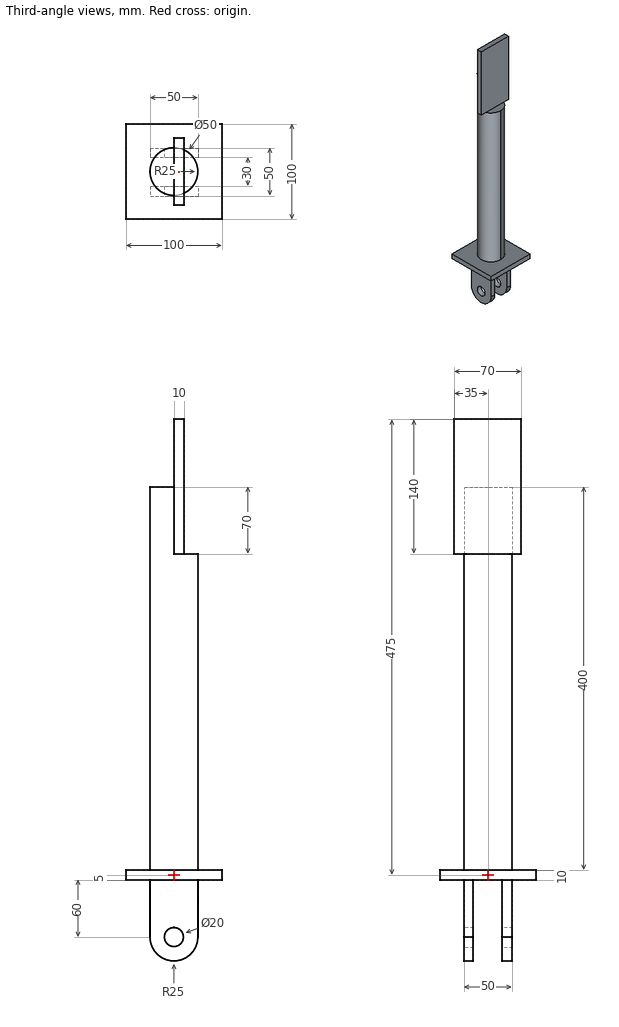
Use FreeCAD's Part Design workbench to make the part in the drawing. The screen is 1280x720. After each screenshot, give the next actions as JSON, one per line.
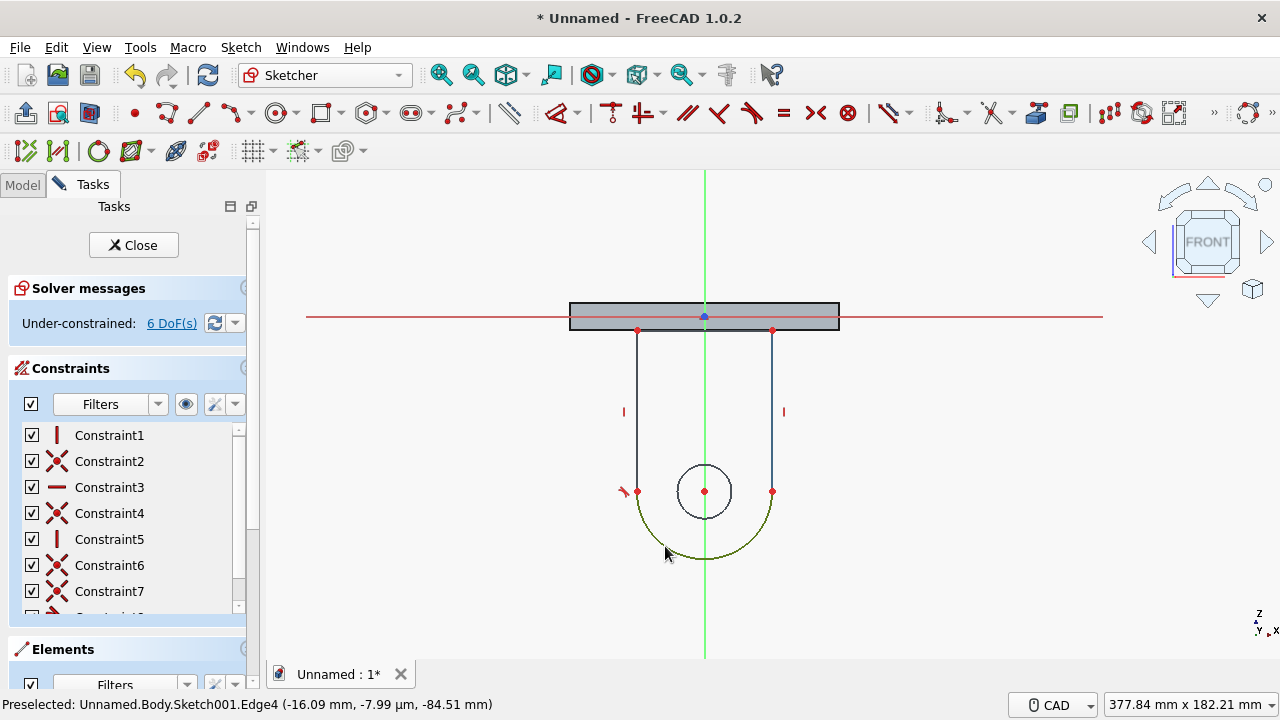
{"action": "key", "text": "t"}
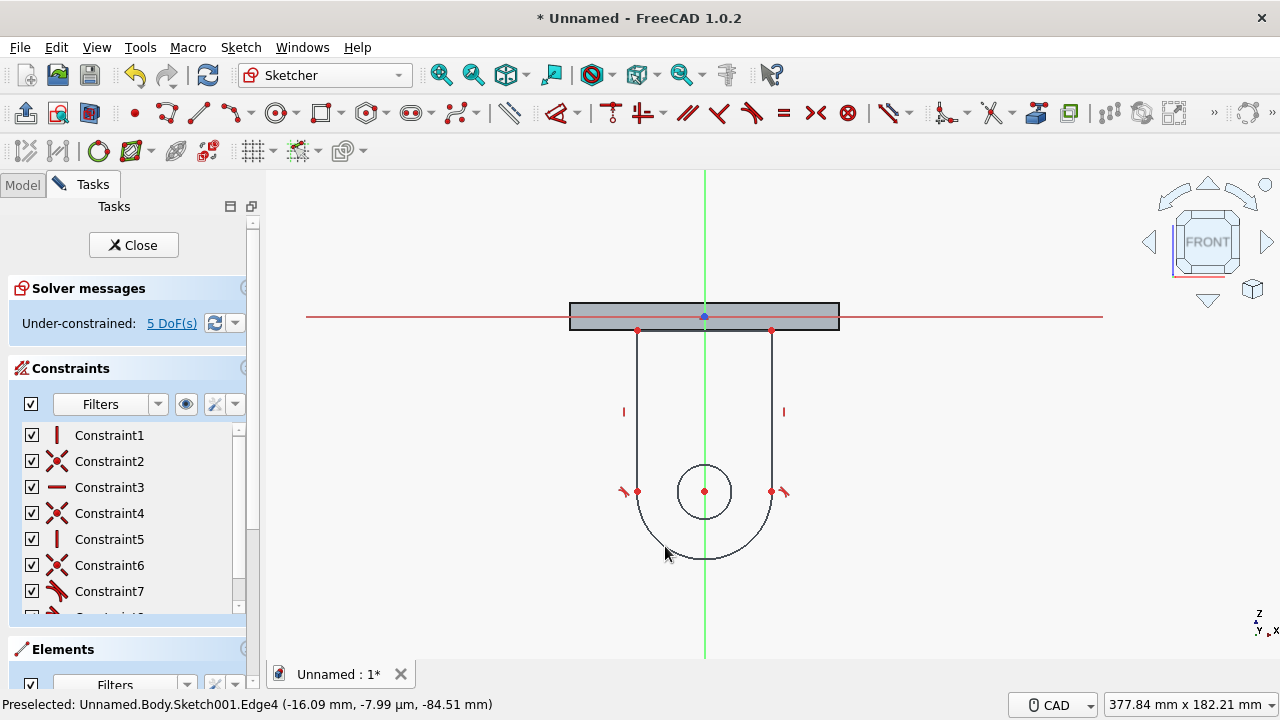
{"action": "left_click", "coordinate": [704, 492]}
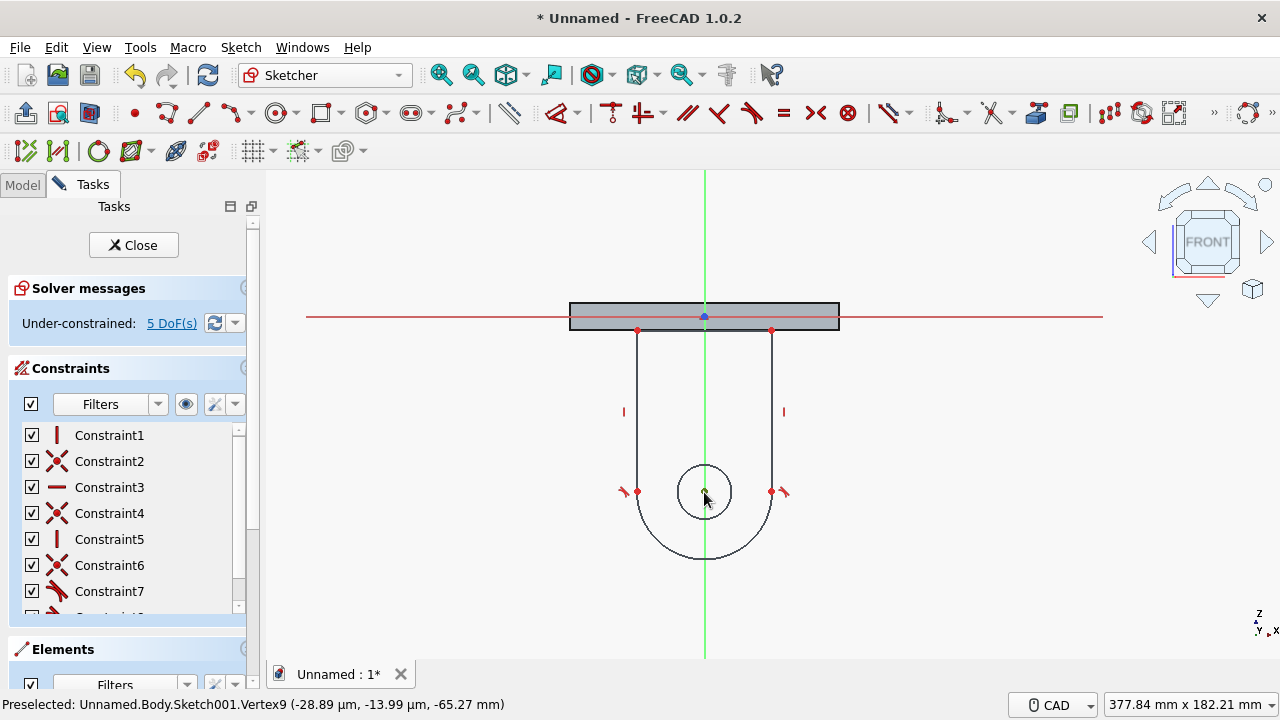
{"action": "left_click", "coordinate": [705, 600]}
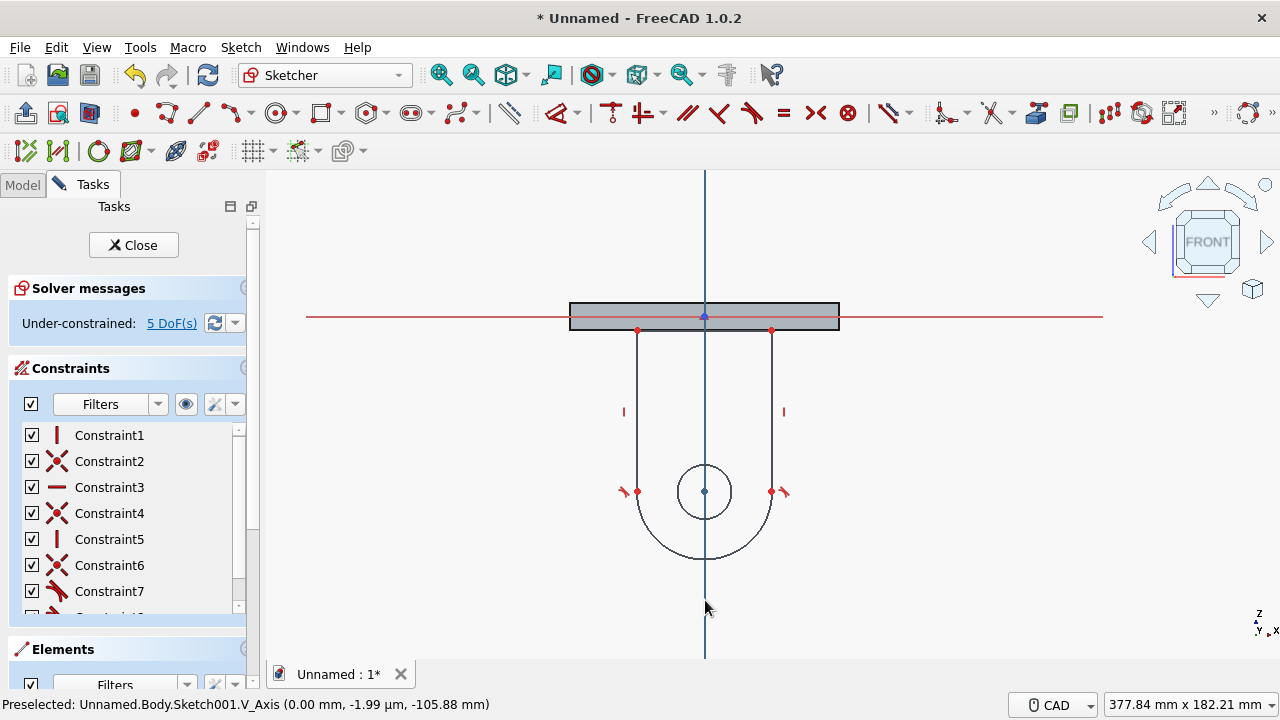
{"action": "key", "text": "c"}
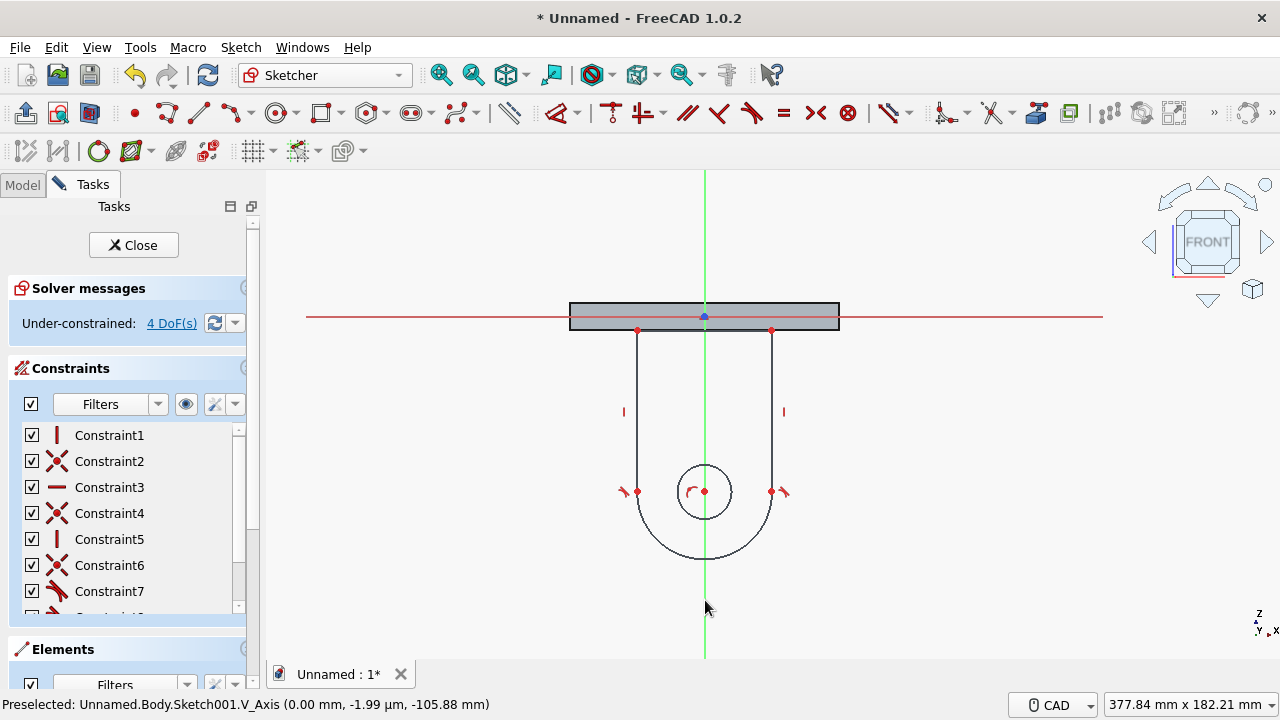
{"action": "key", "text": "d"}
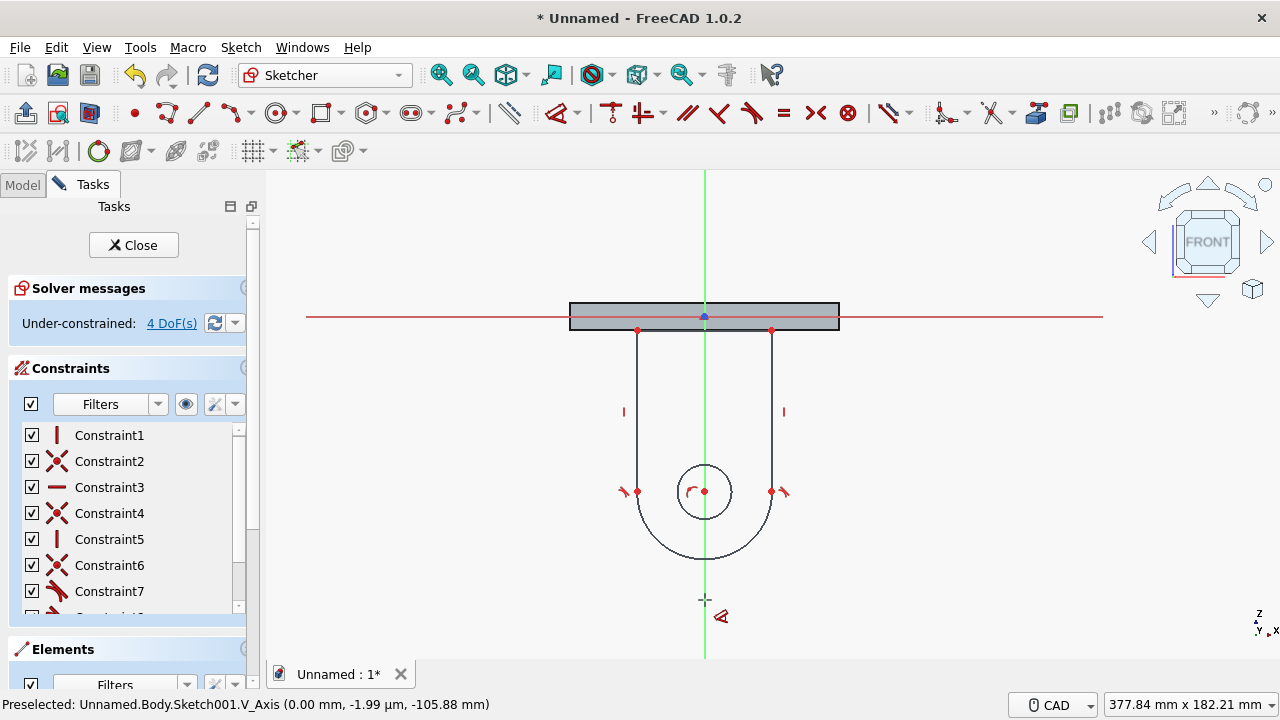
{"action": "left_click", "coordinate": [665, 547]}
{"action": "left_click", "coordinate": [646, 573]}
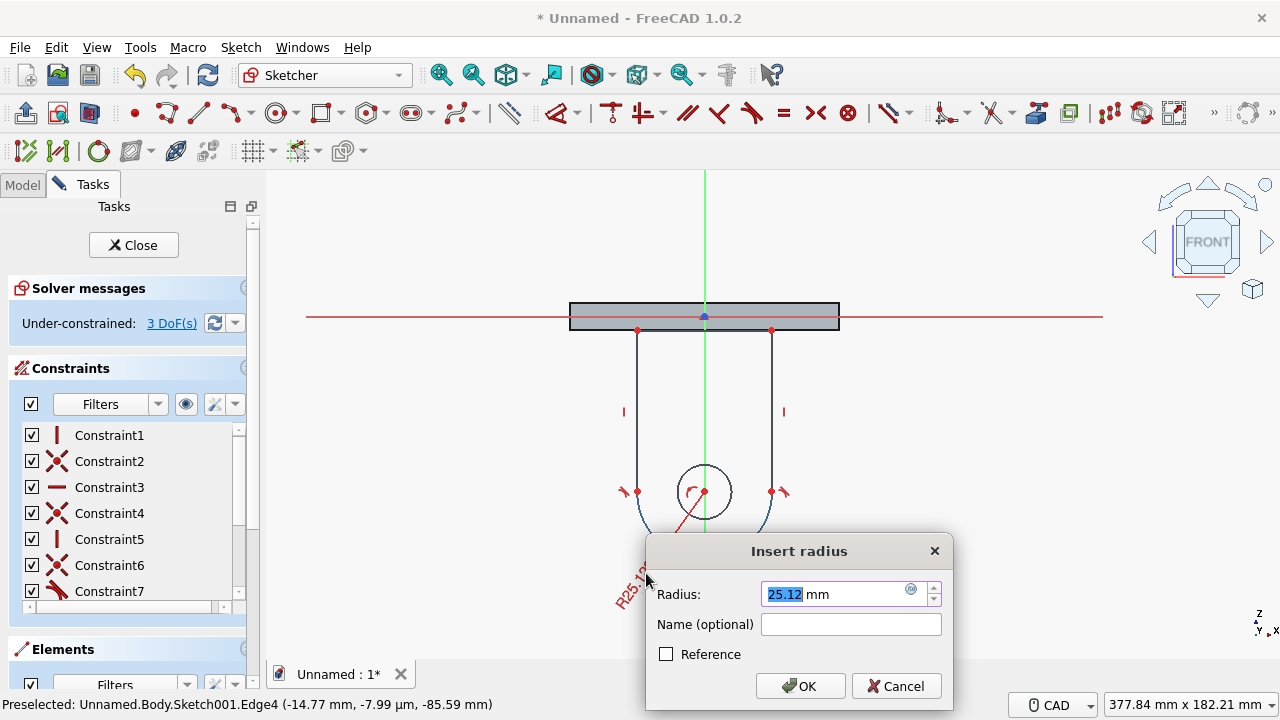
{"action": "type", "text": "25"}
{"action": "key", "text": "Return"}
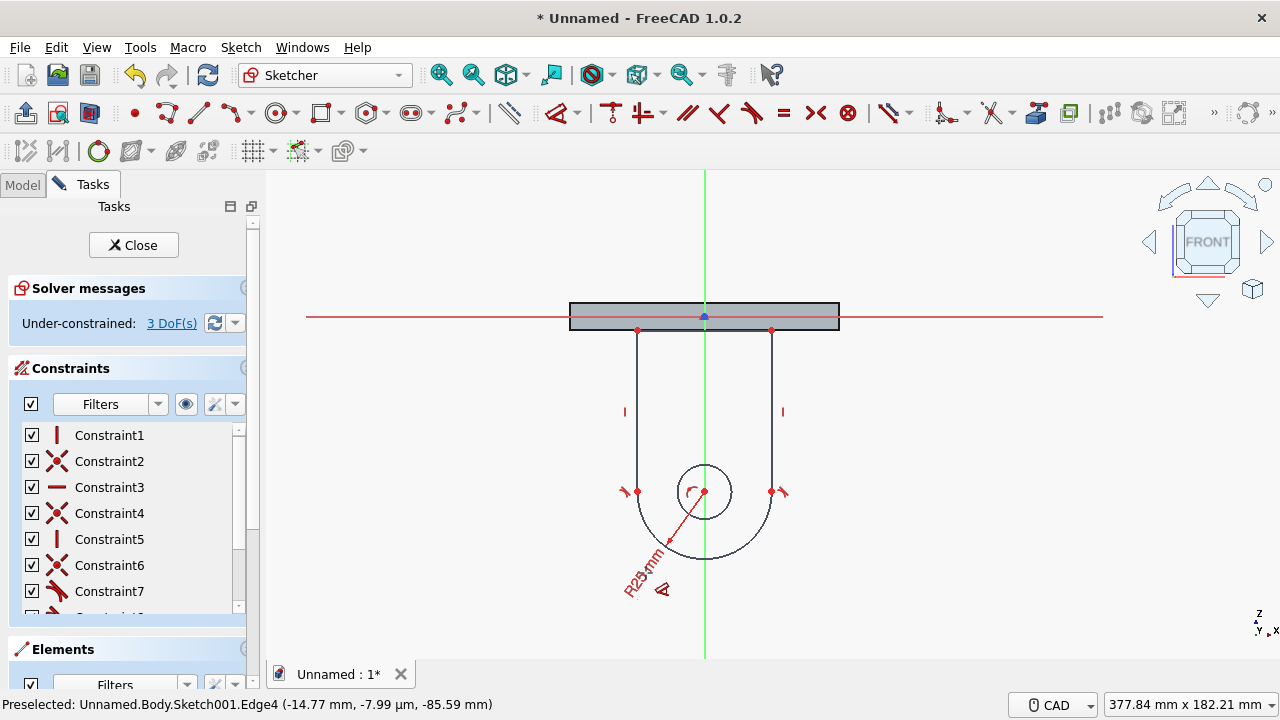
{"action": "left_click", "coordinate": [724, 473]}
{"action": "left_click", "coordinate": [747, 451]}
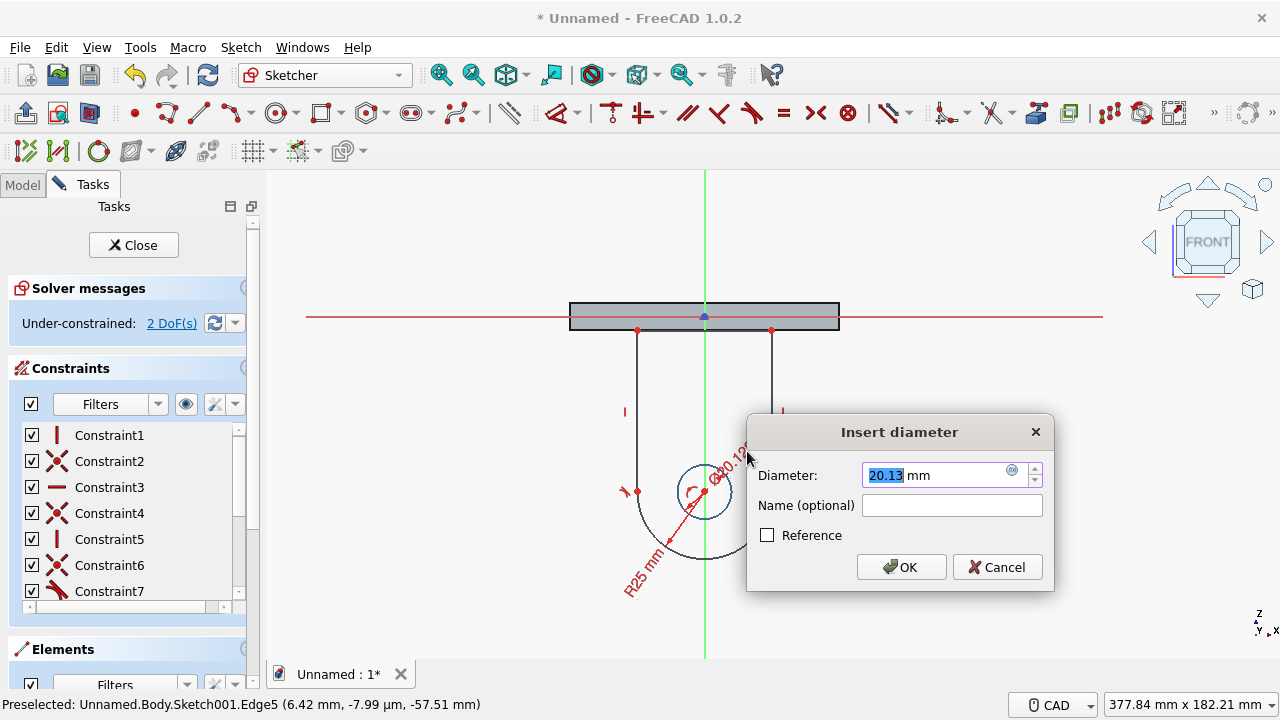
{"action": "type", "text": "20"}
{"action": "key", "text": "Return"}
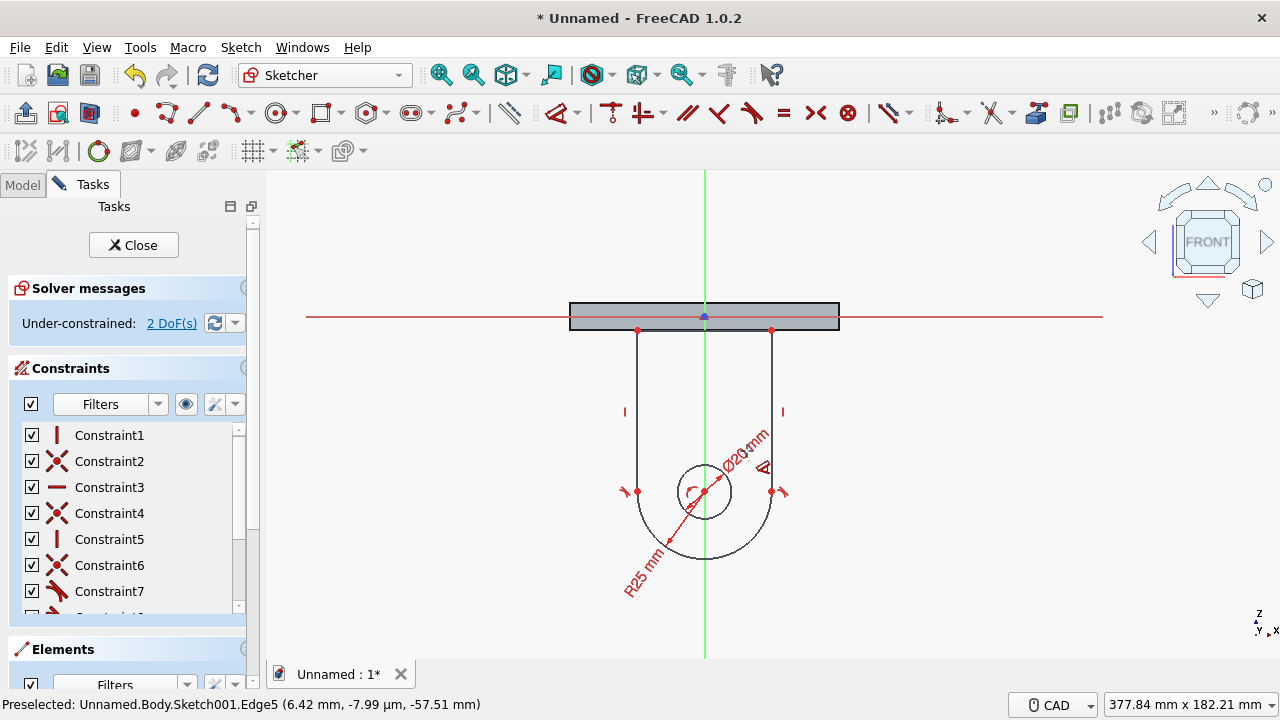
{"action": "left_click", "coordinate": [637, 444]}
{"action": "left_click", "coordinate": [603, 411]}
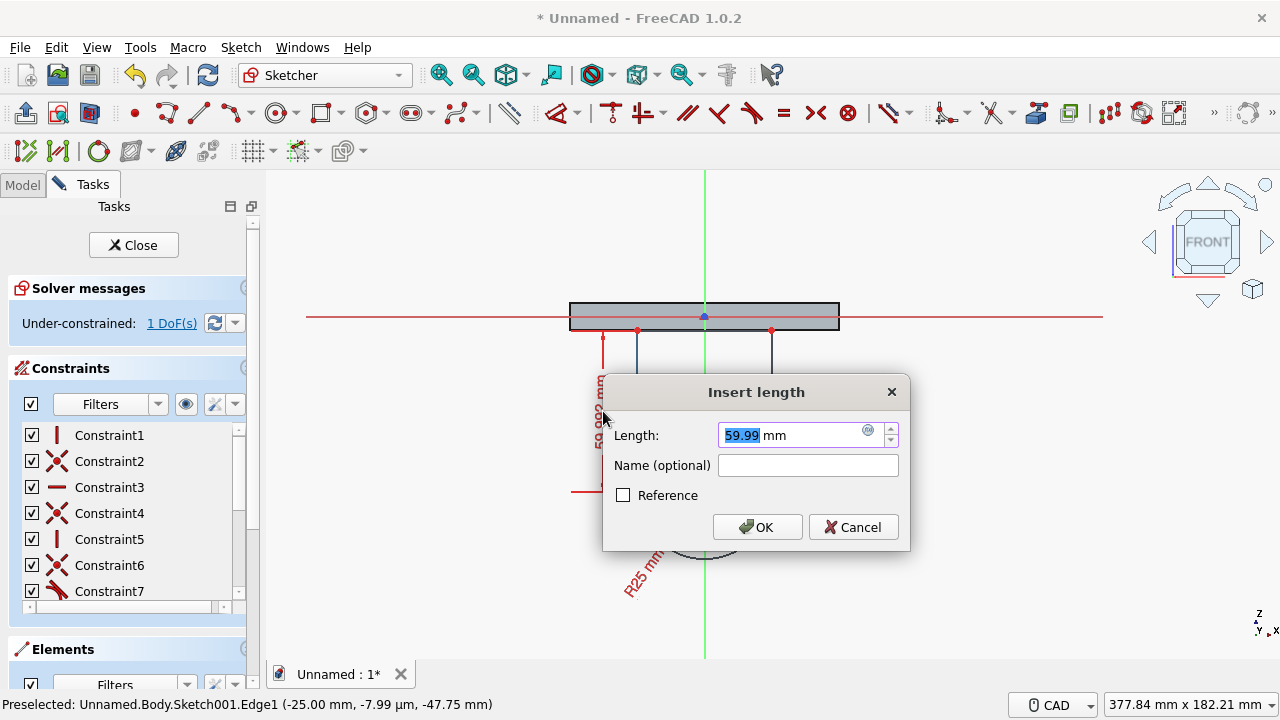
{"action": "type", "text": "60"}
{"action": "key", "text": "Return"}